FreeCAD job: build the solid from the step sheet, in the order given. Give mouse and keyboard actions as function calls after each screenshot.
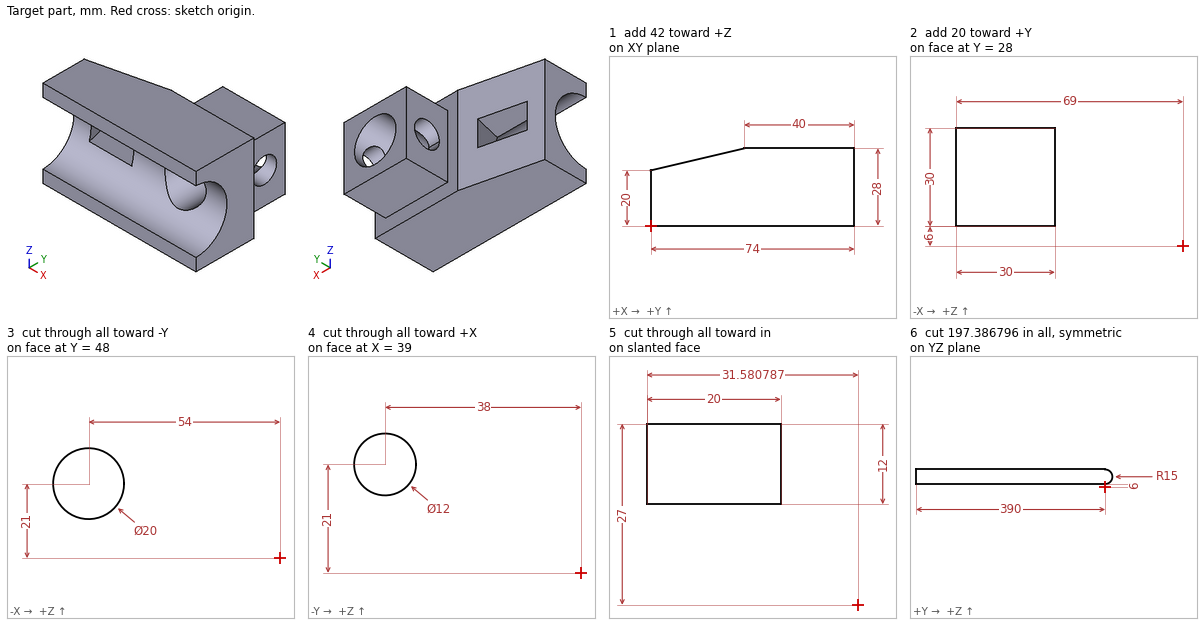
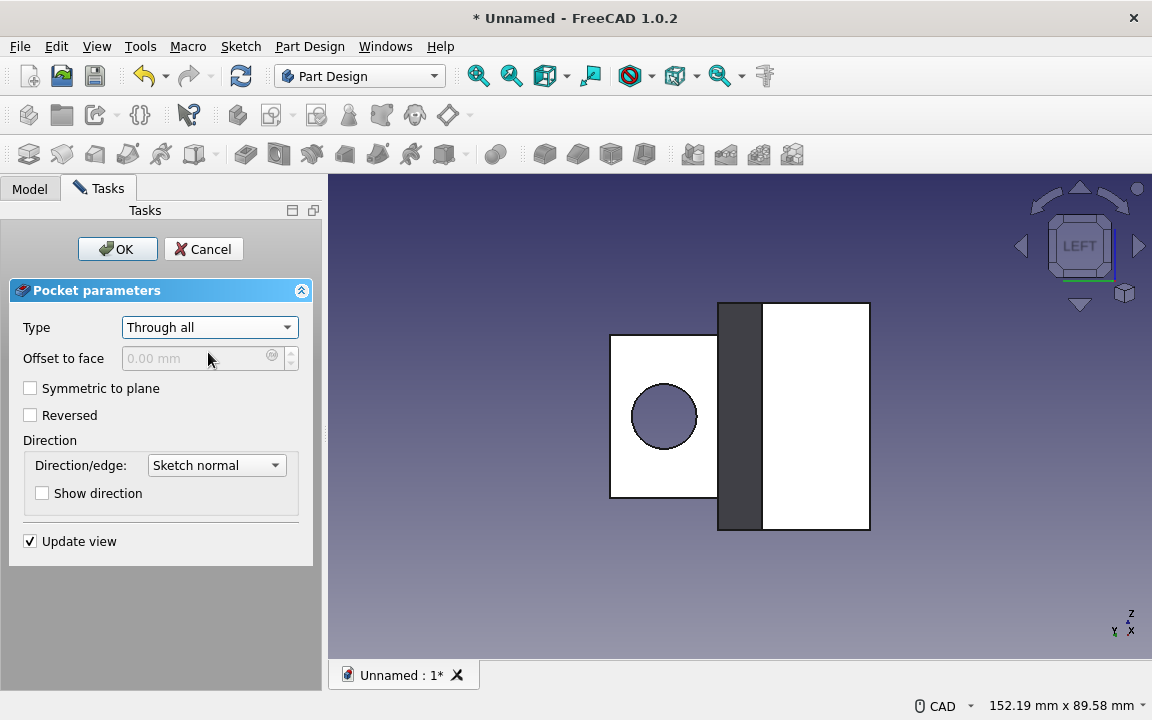
click(118, 249)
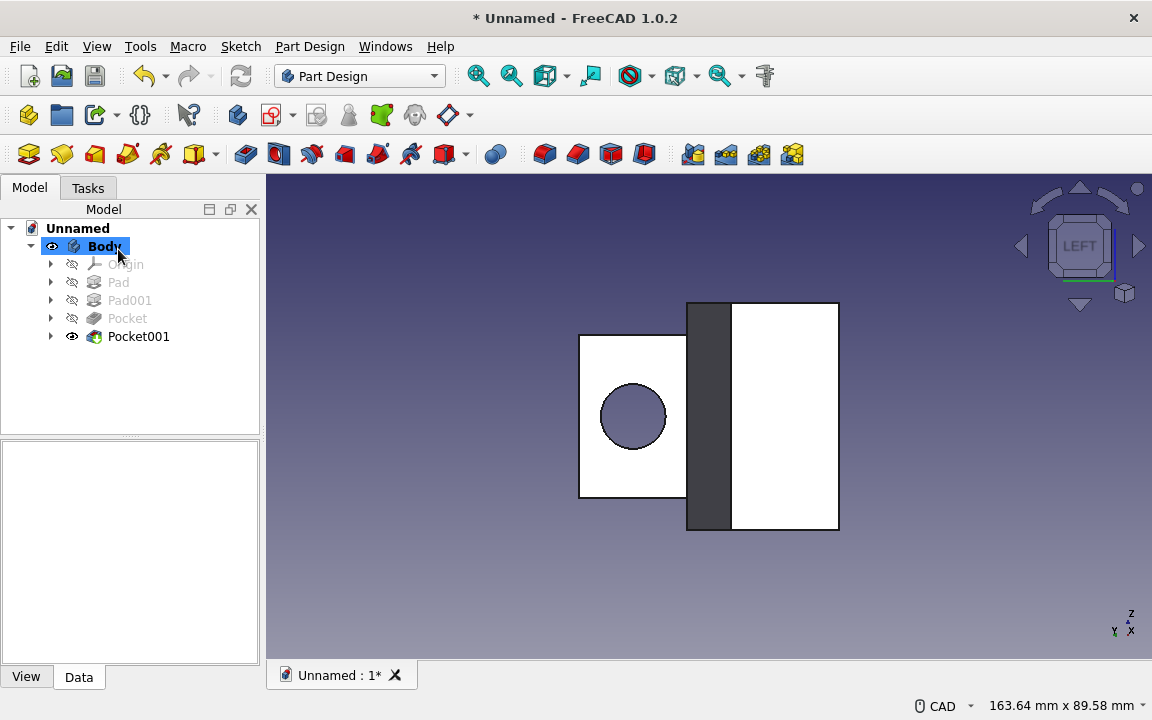
click(709, 416)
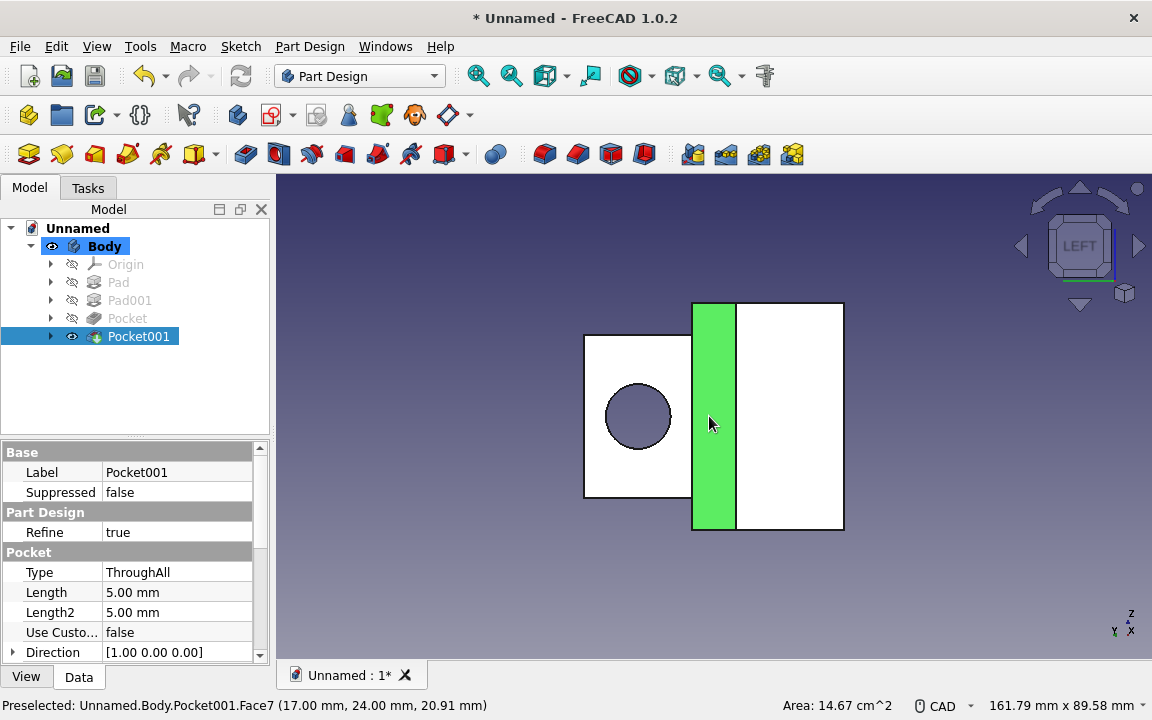
click(270, 116)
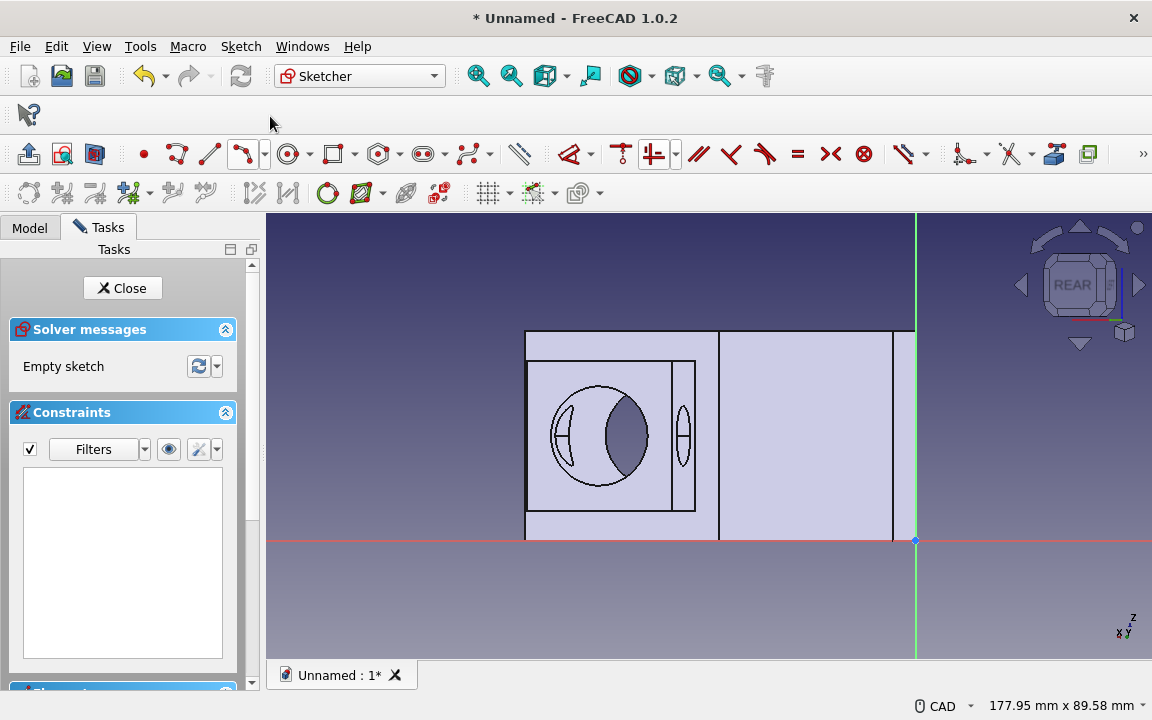
scroll(987, 504, up, 4)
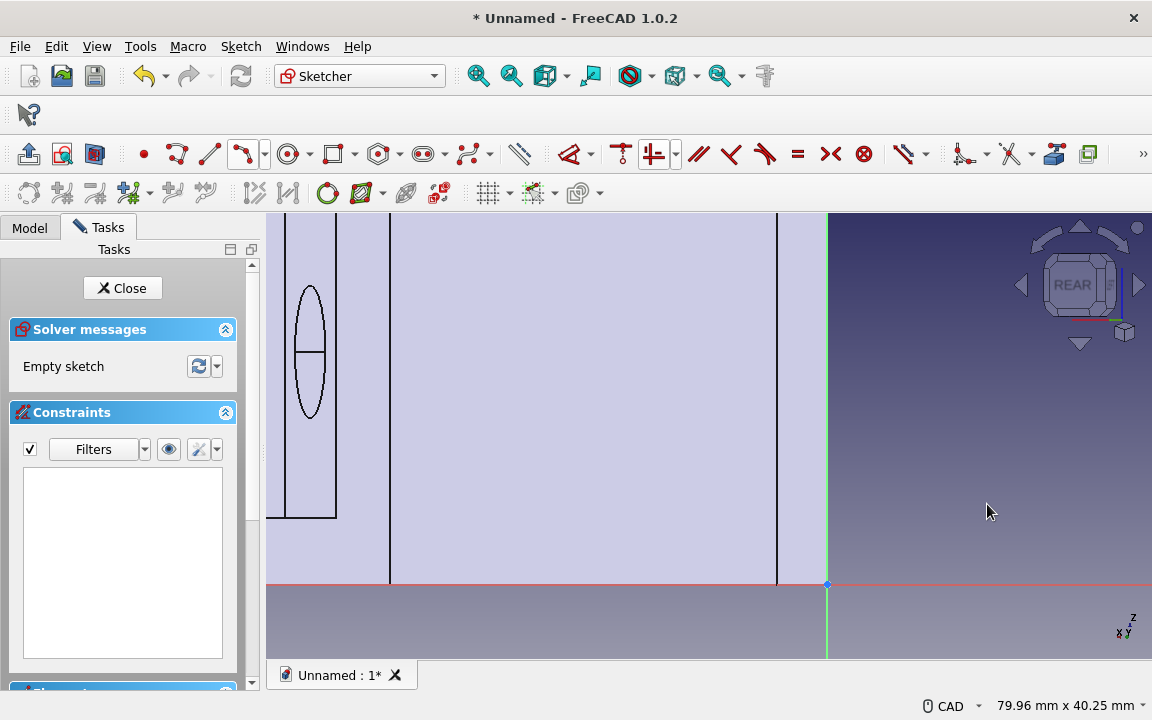
click(332, 154)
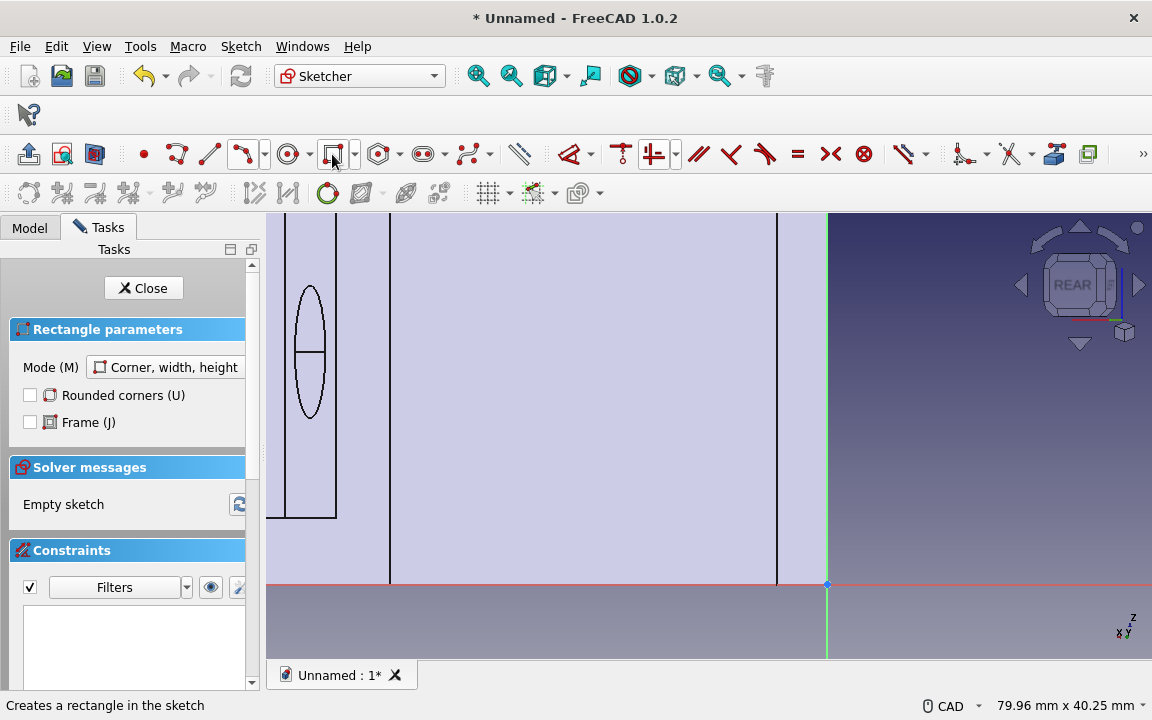
click(477, 285)
move(699, 418)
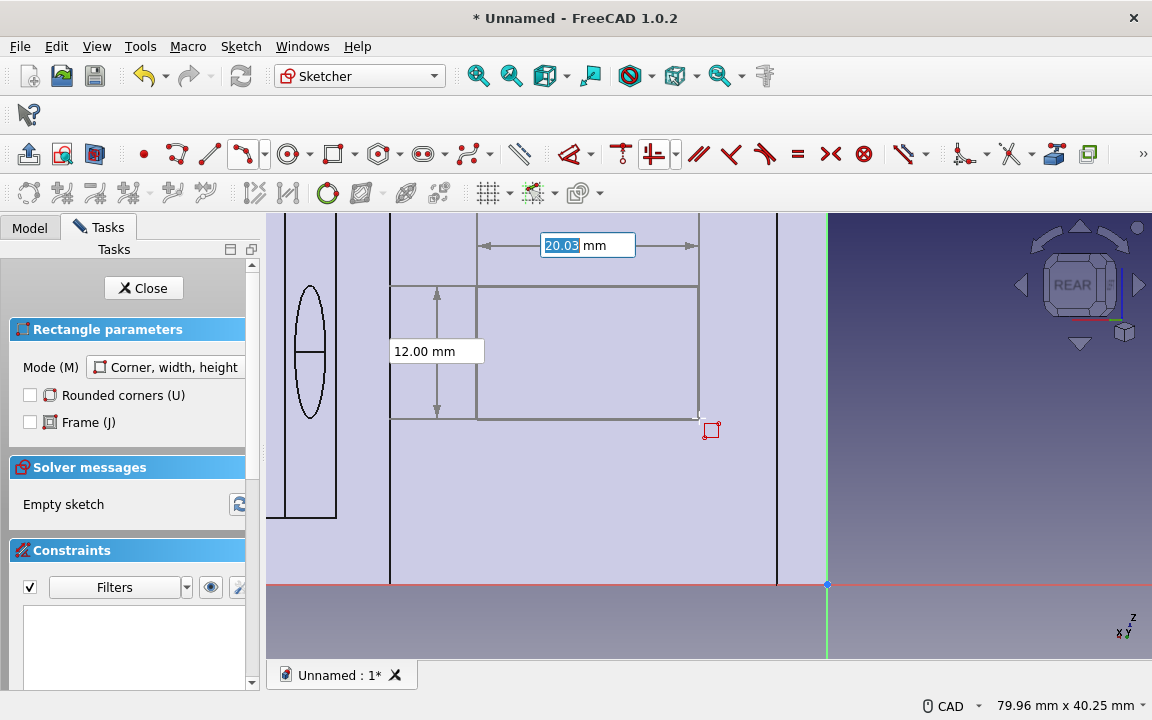
text(20)
key(Tab)
text(12)
key(Return)
key(Escape)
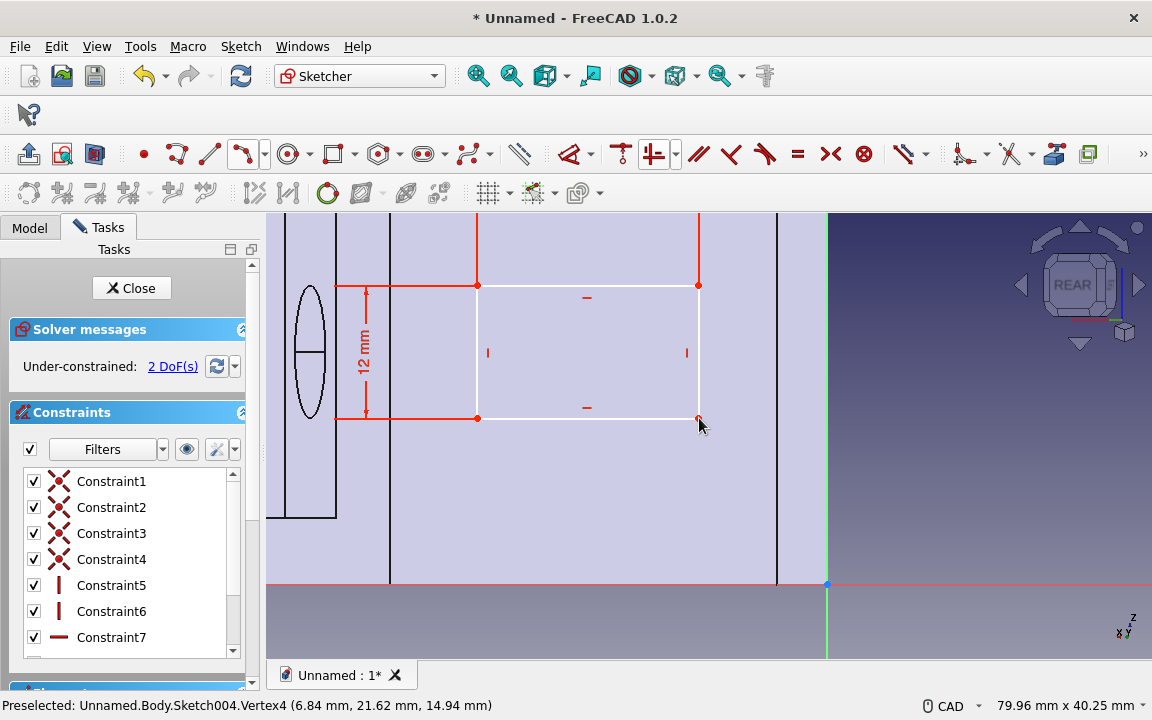
click(568, 154)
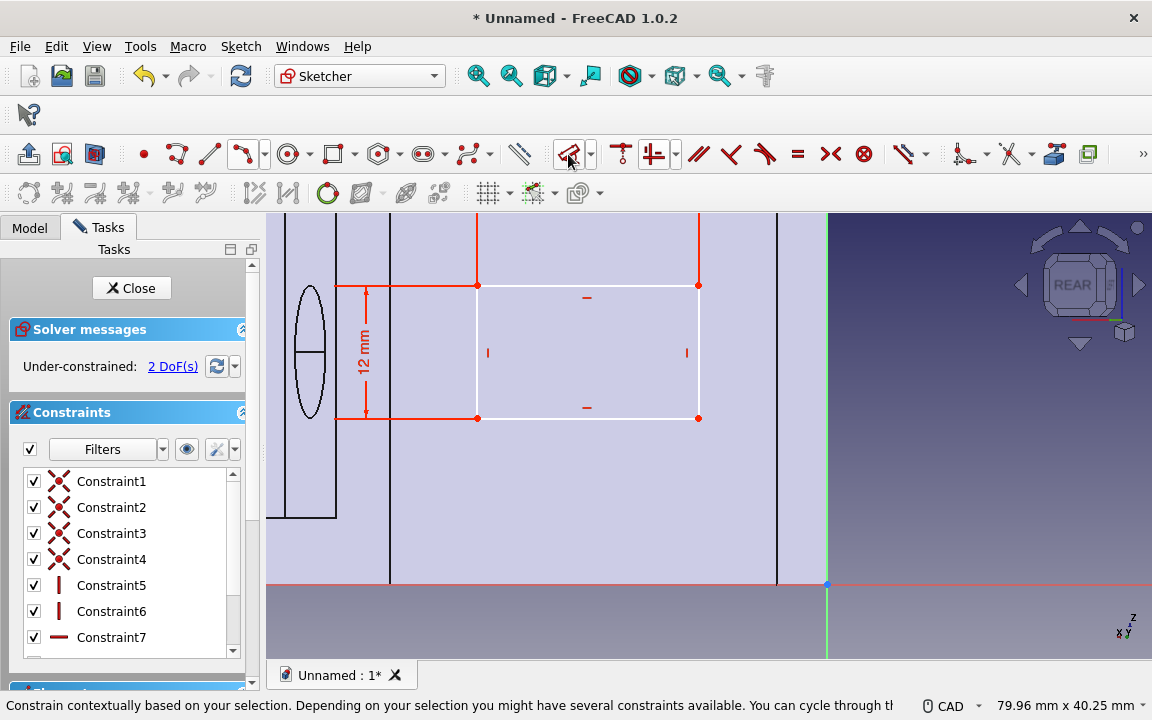
click(477, 286)
click(443, 435)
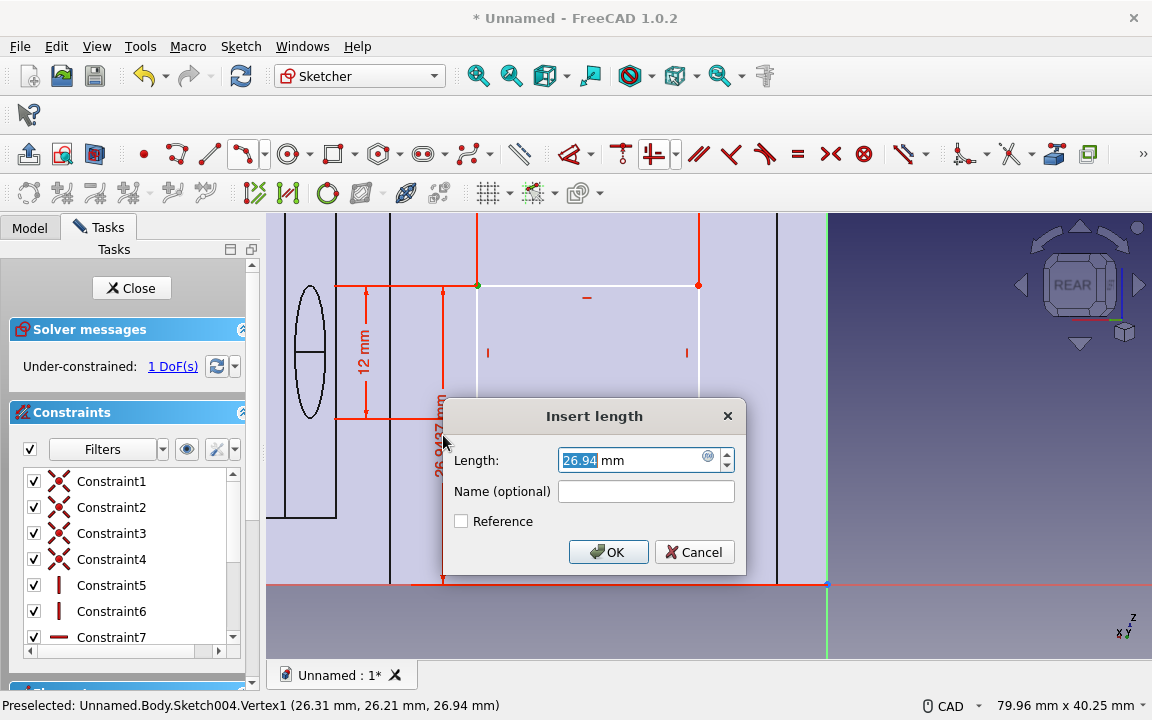
text(27)
key(Return)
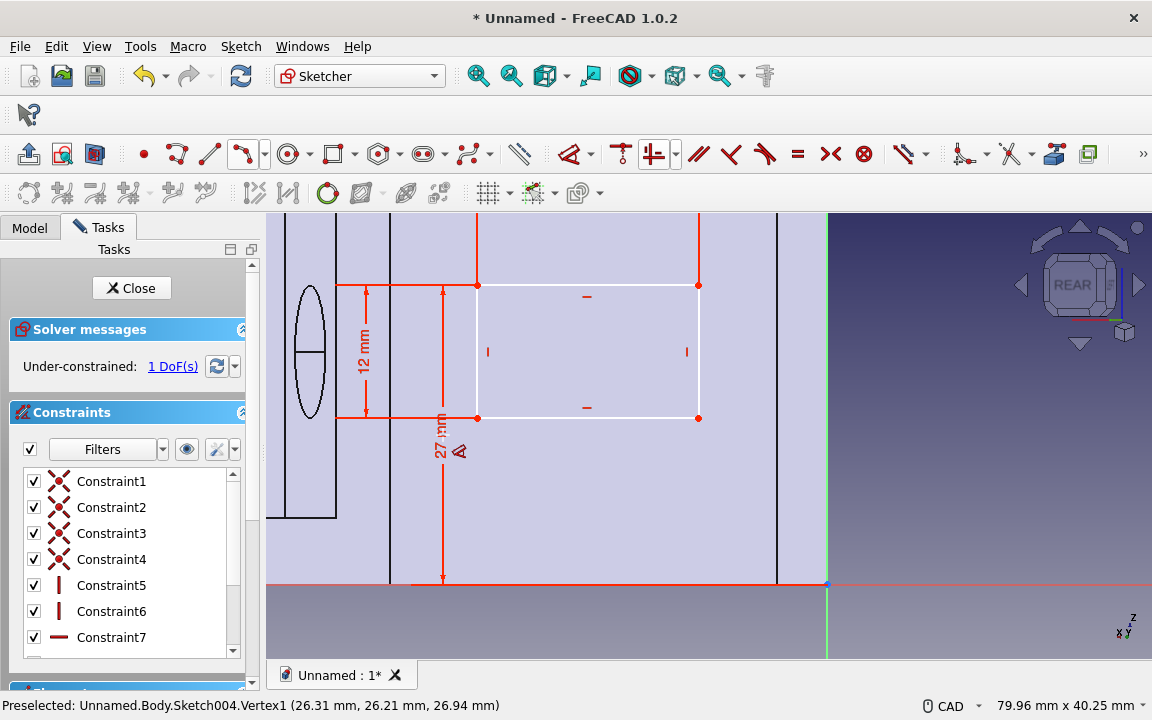
click(477, 285)
click(652, 251)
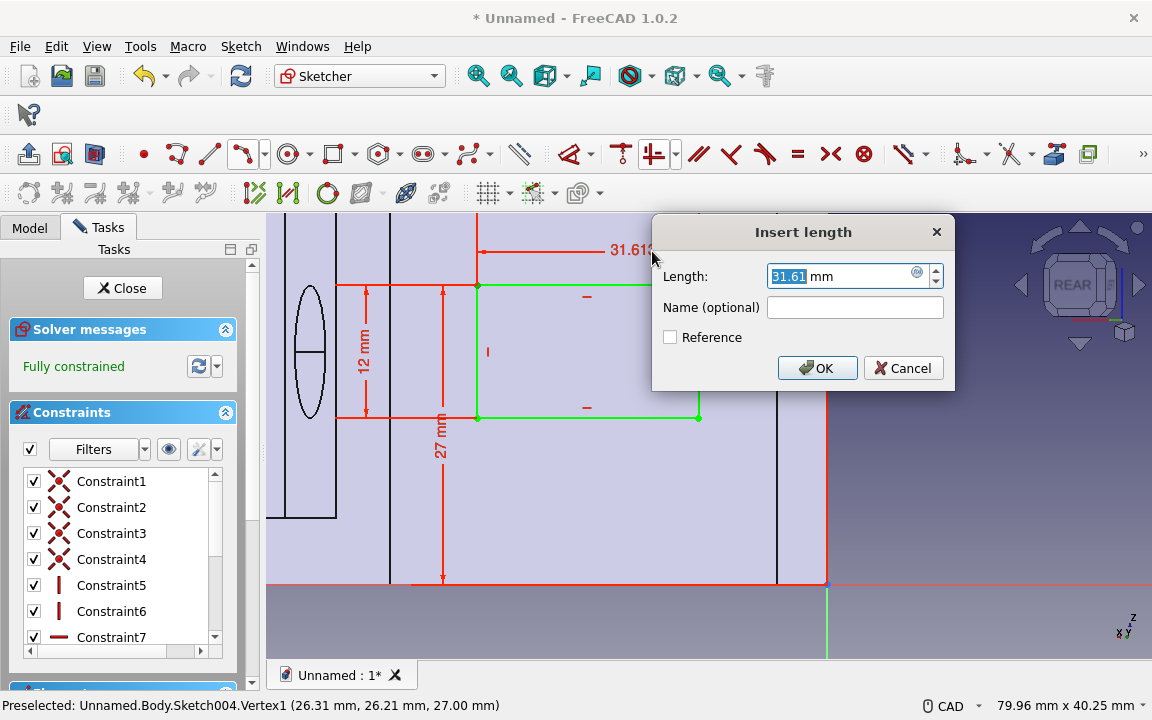
text(31.580787)
key(Return)
key(Escape)